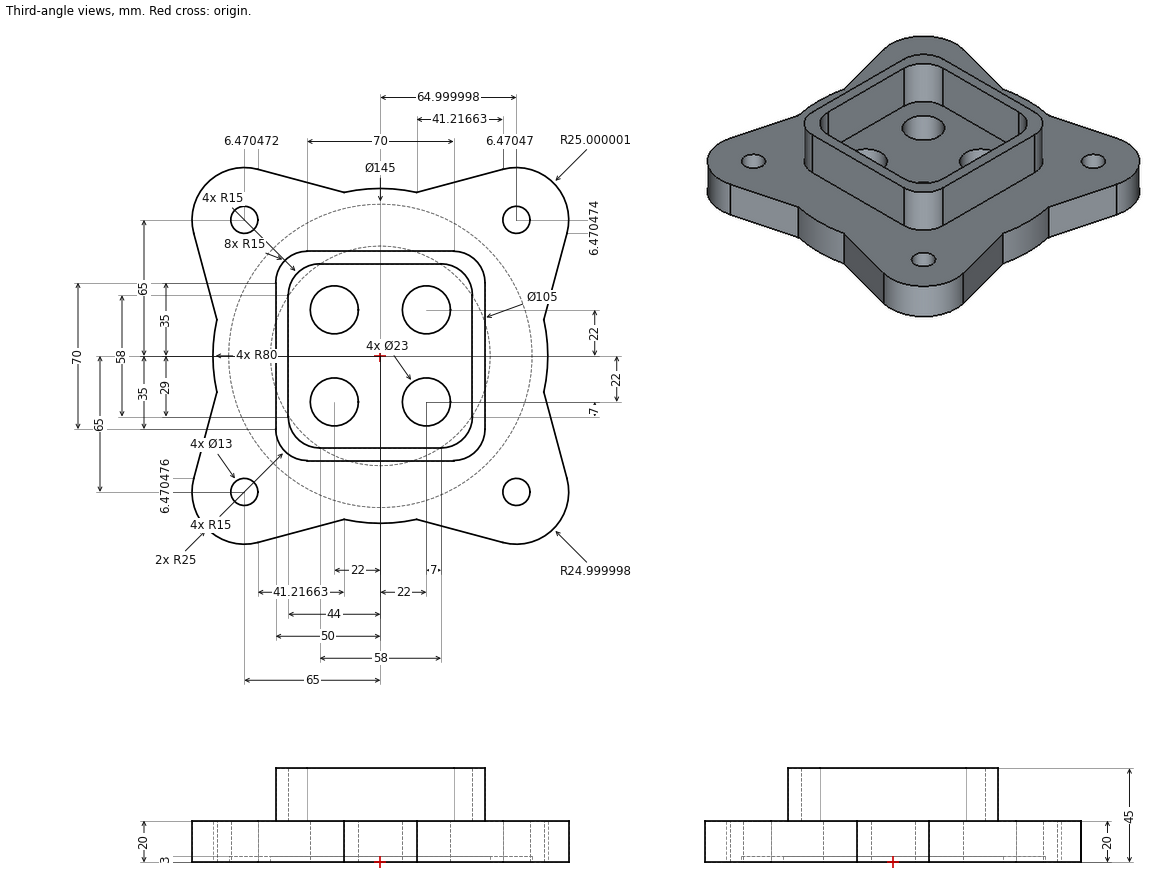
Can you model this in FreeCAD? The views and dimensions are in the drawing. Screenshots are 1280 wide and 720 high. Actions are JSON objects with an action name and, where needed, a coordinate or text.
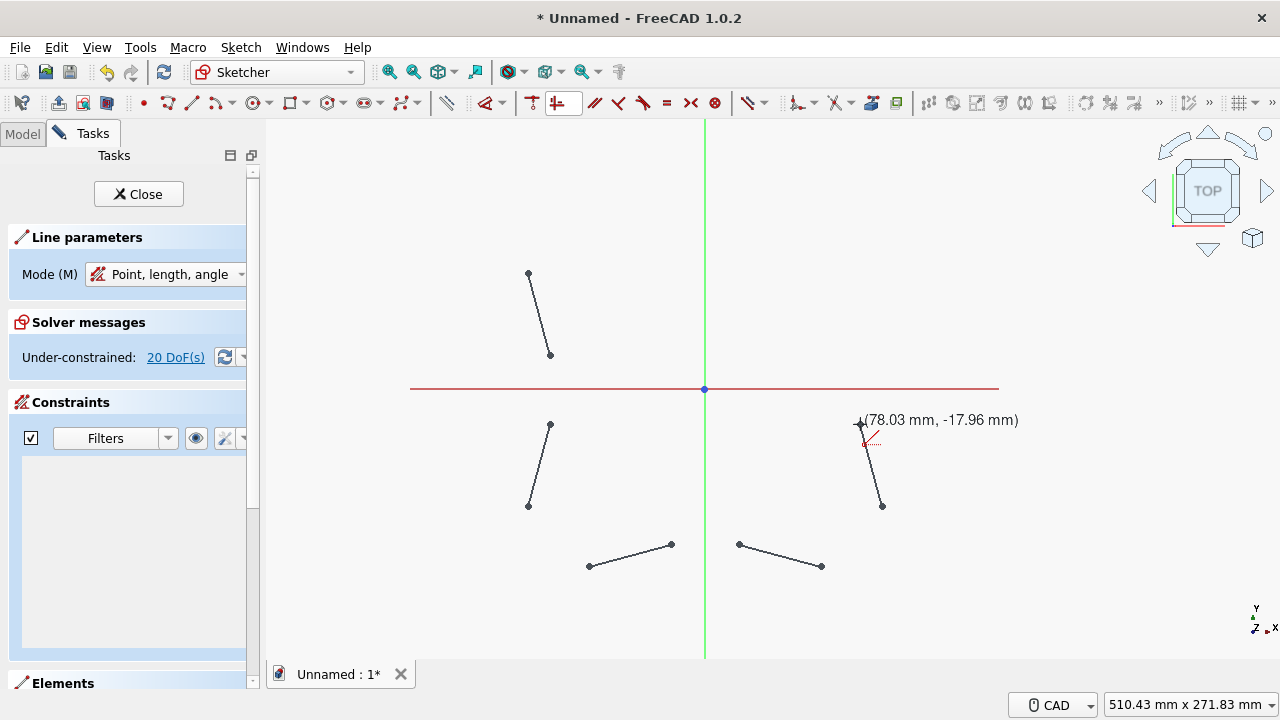
{"action": "left_click", "coordinate": [860, 355]}
{"action": "left_click", "coordinate": [882, 273]}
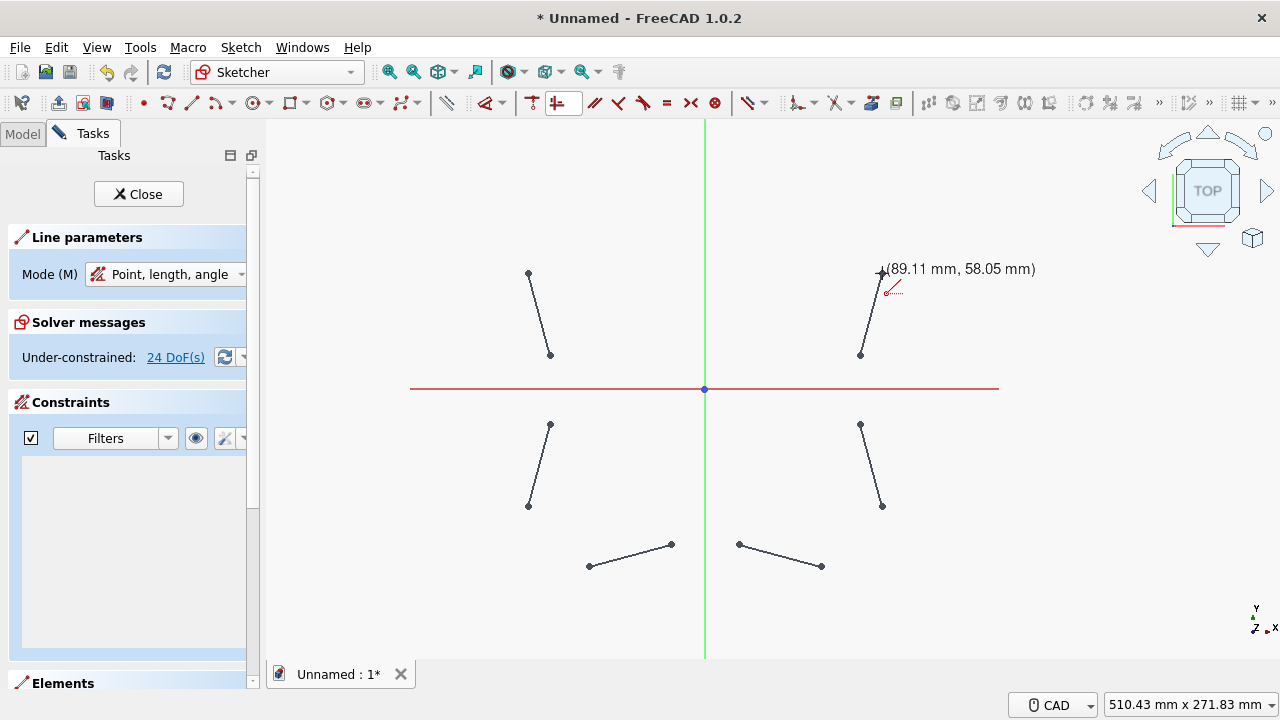
{"action": "left_click", "coordinate": [821, 212]}
{"action": "left_click", "coordinate": [739, 234]}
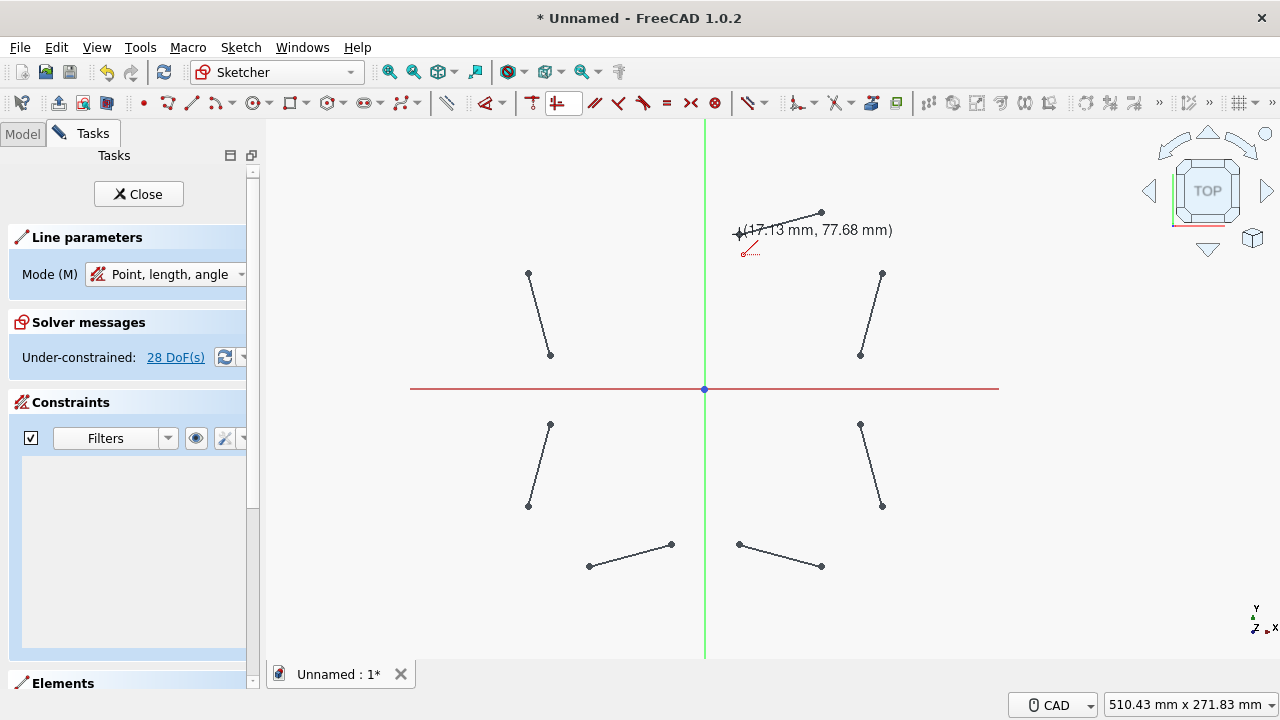
{"action": "left_click", "coordinate": [671, 234]}
{"action": "left_click", "coordinate": [589, 212]}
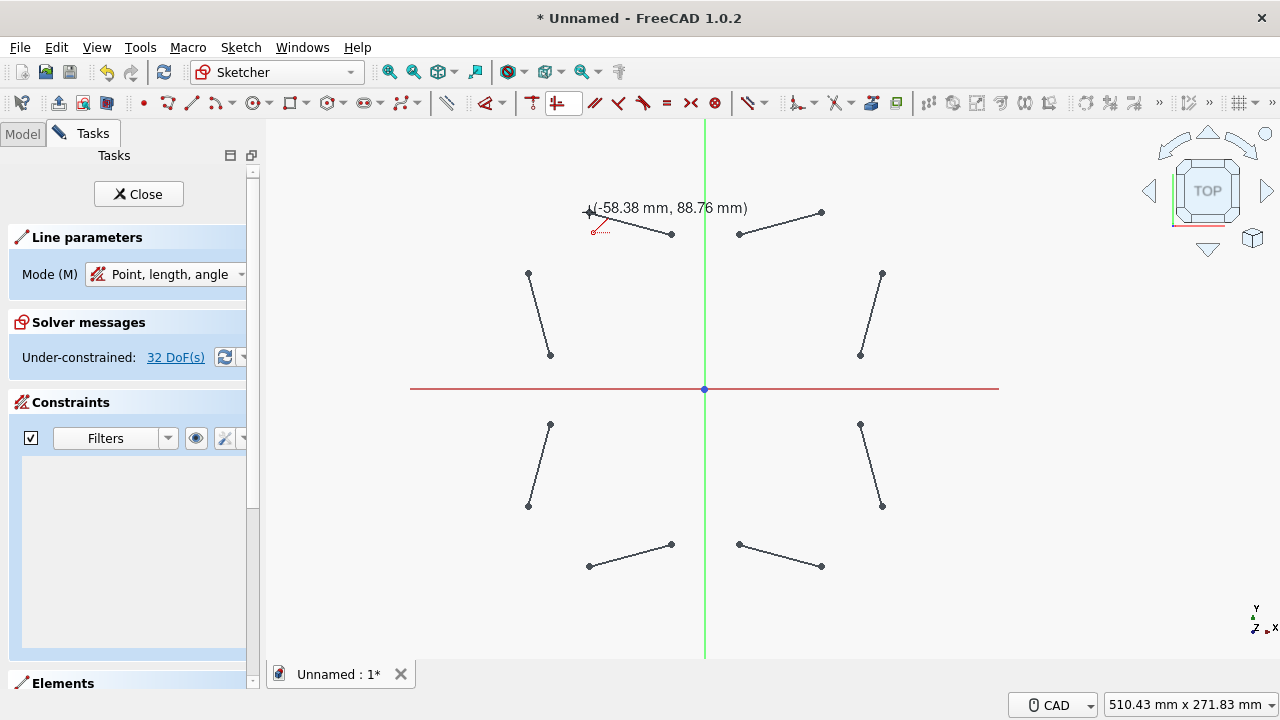
{"action": "left_click", "coordinate": [234, 104]}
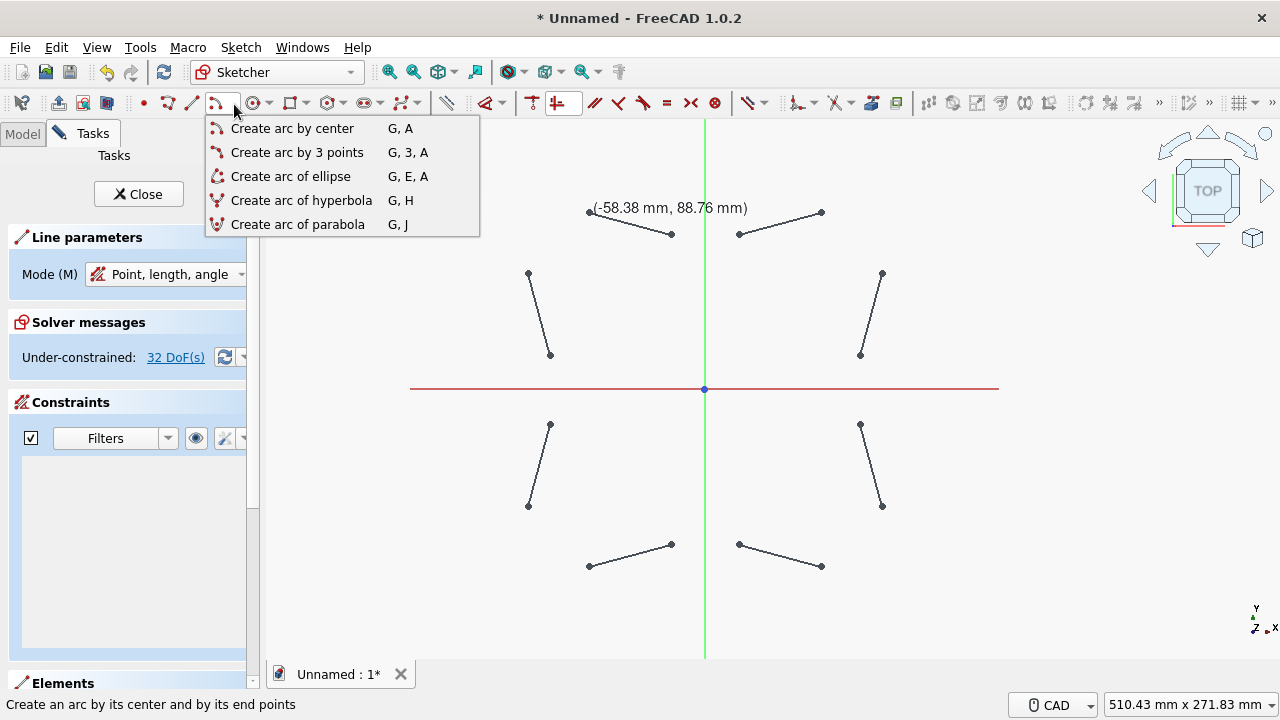
{"action": "left_click", "coordinate": [342, 152]}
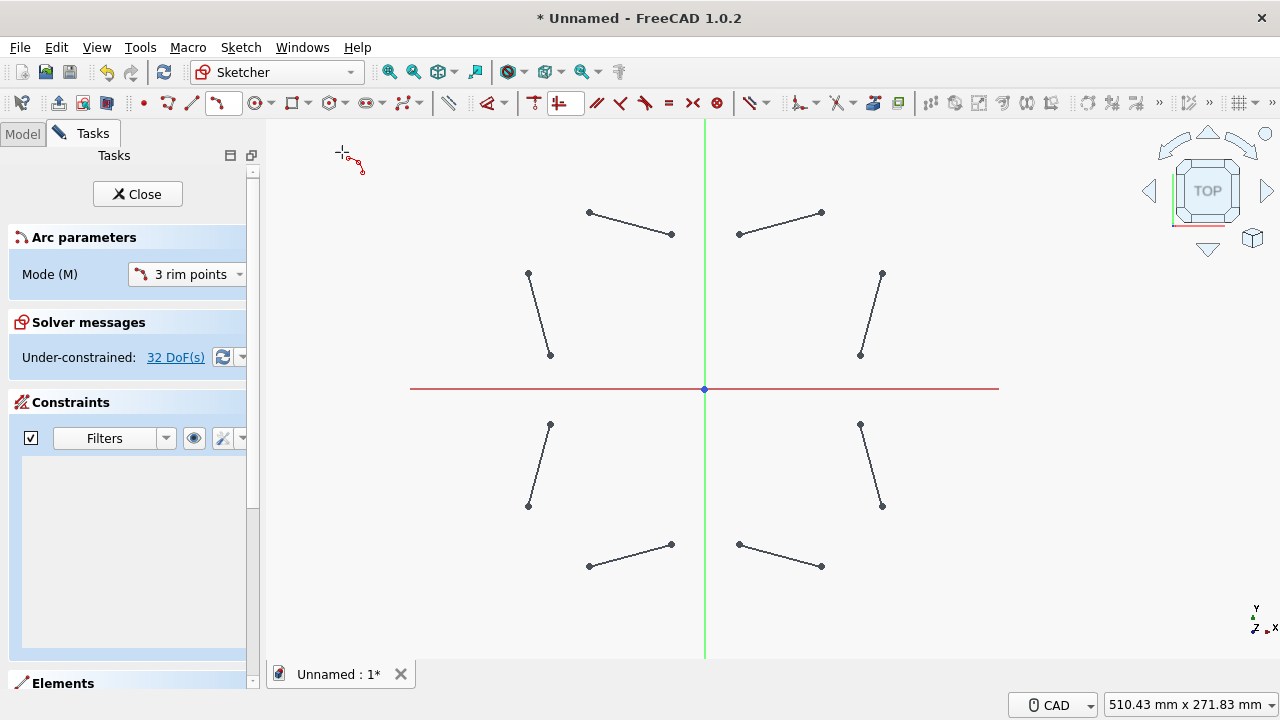
{"action": "left_click", "coordinate": [550, 356]}
{"action": "left_click", "coordinate": [550, 425]}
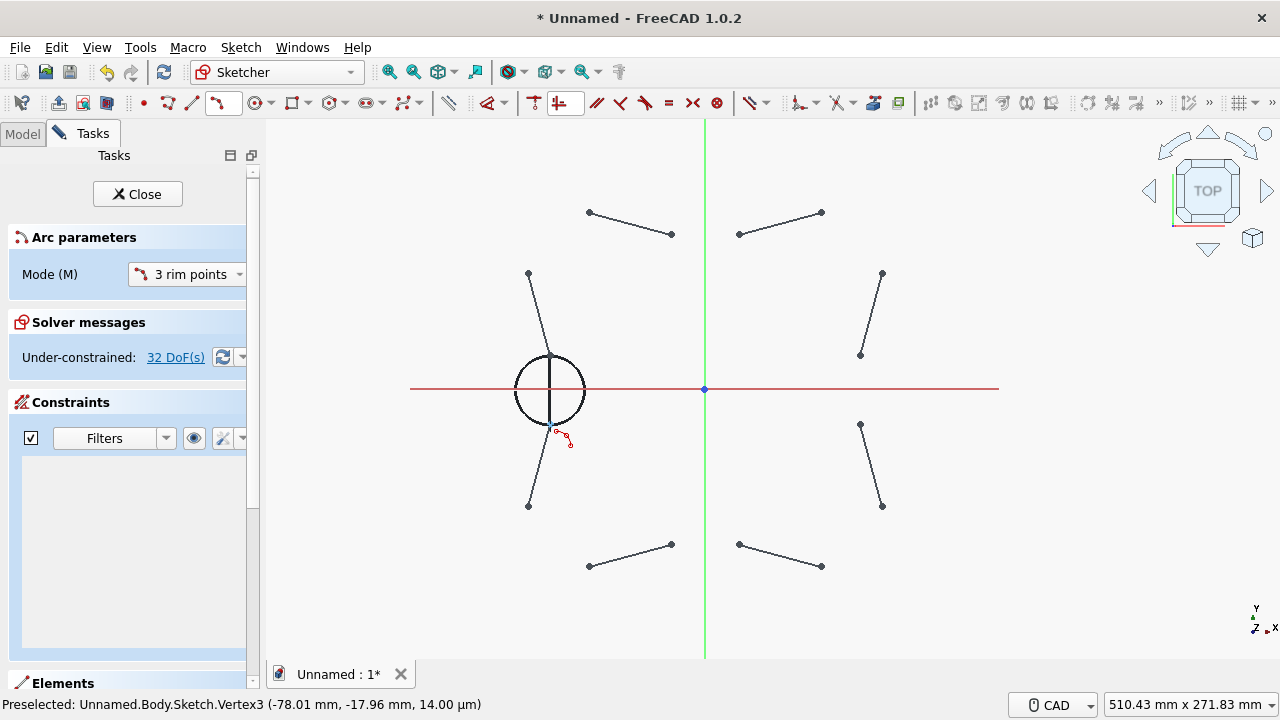
{"action": "scroll", "coordinate": [546, 382], "scroll_direction": "up", "scroll_amount": 8}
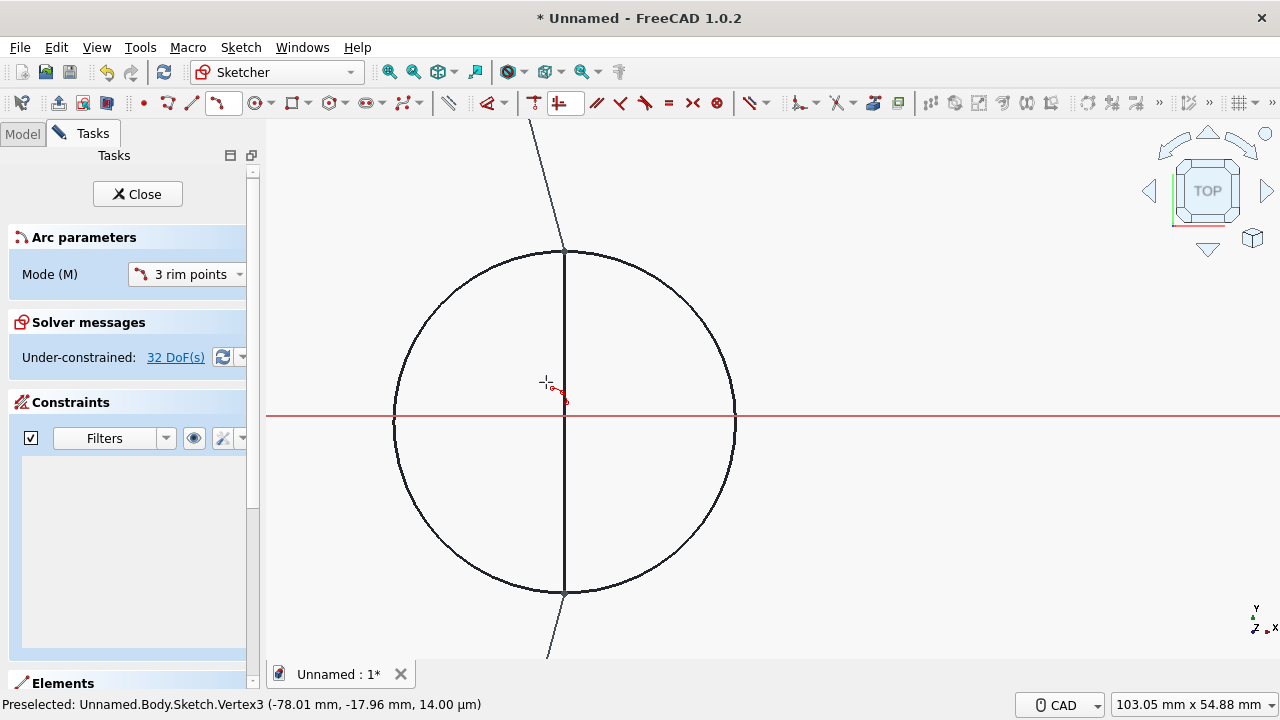
{"action": "left_click", "coordinate": [546, 382]}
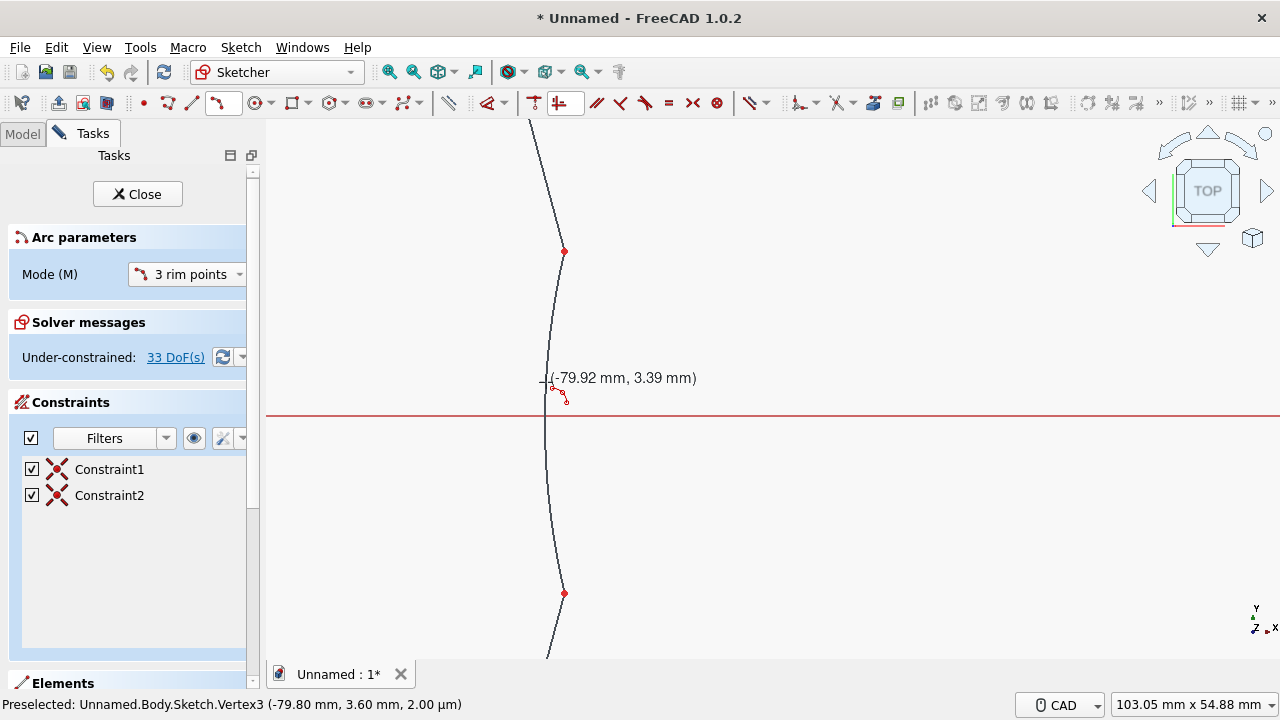
{"action": "scroll", "coordinate": [546, 382], "scroll_direction": "down", "scroll_amount": 8}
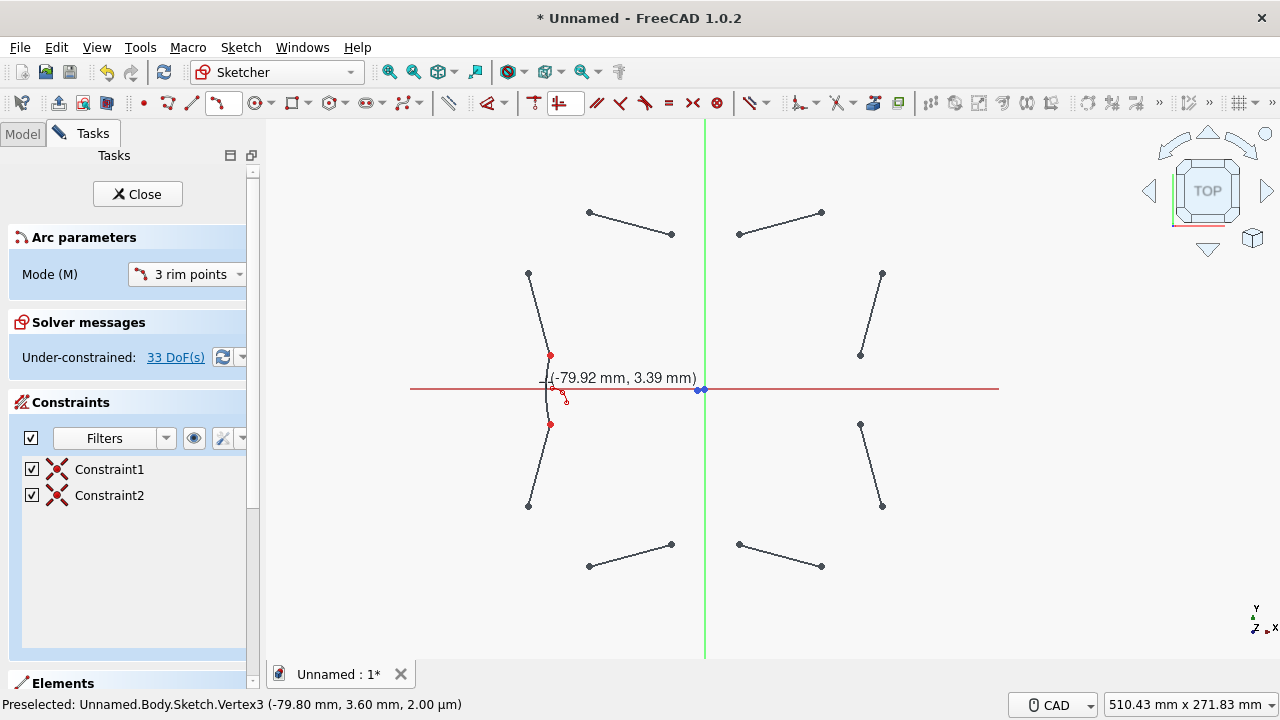
{"action": "left_click", "coordinate": [528, 507]}
{"action": "left_click", "coordinate": [589, 567]}
{"action": "left_click", "coordinate": [541, 554]}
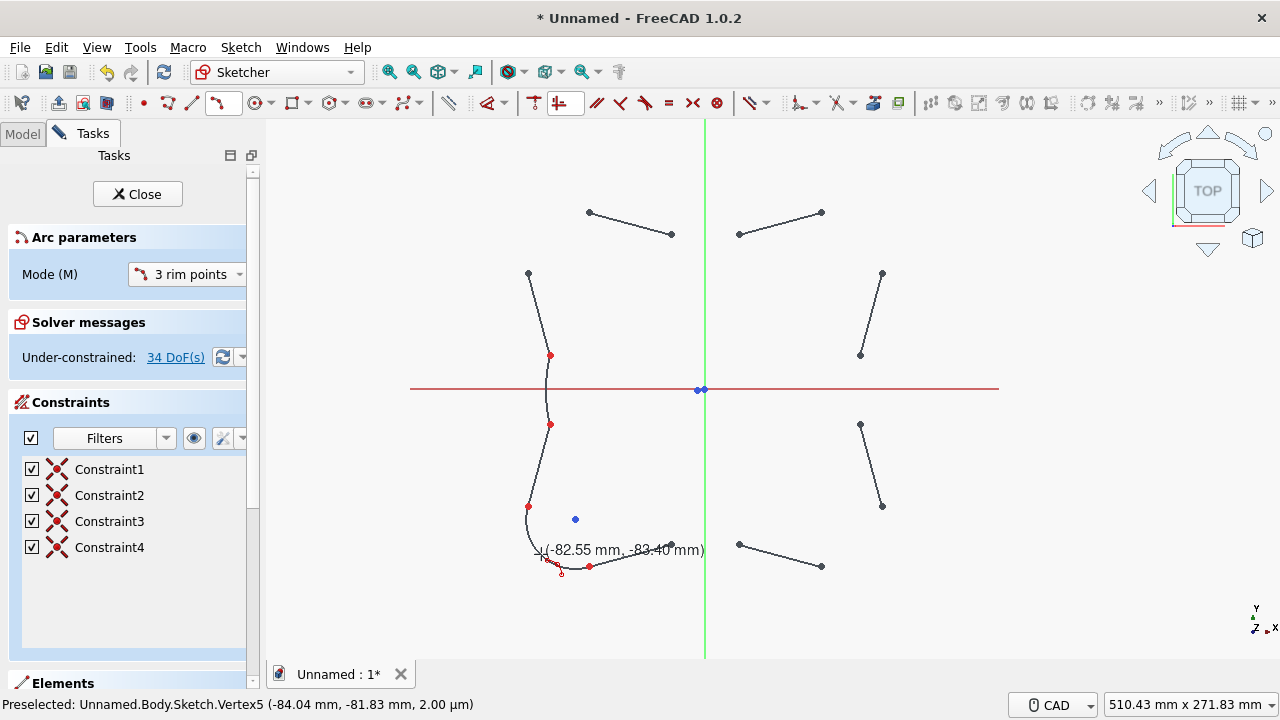
{"action": "left_click", "coordinate": [671, 545]}
{"action": "left_click", "coordinate": [739, 545]}